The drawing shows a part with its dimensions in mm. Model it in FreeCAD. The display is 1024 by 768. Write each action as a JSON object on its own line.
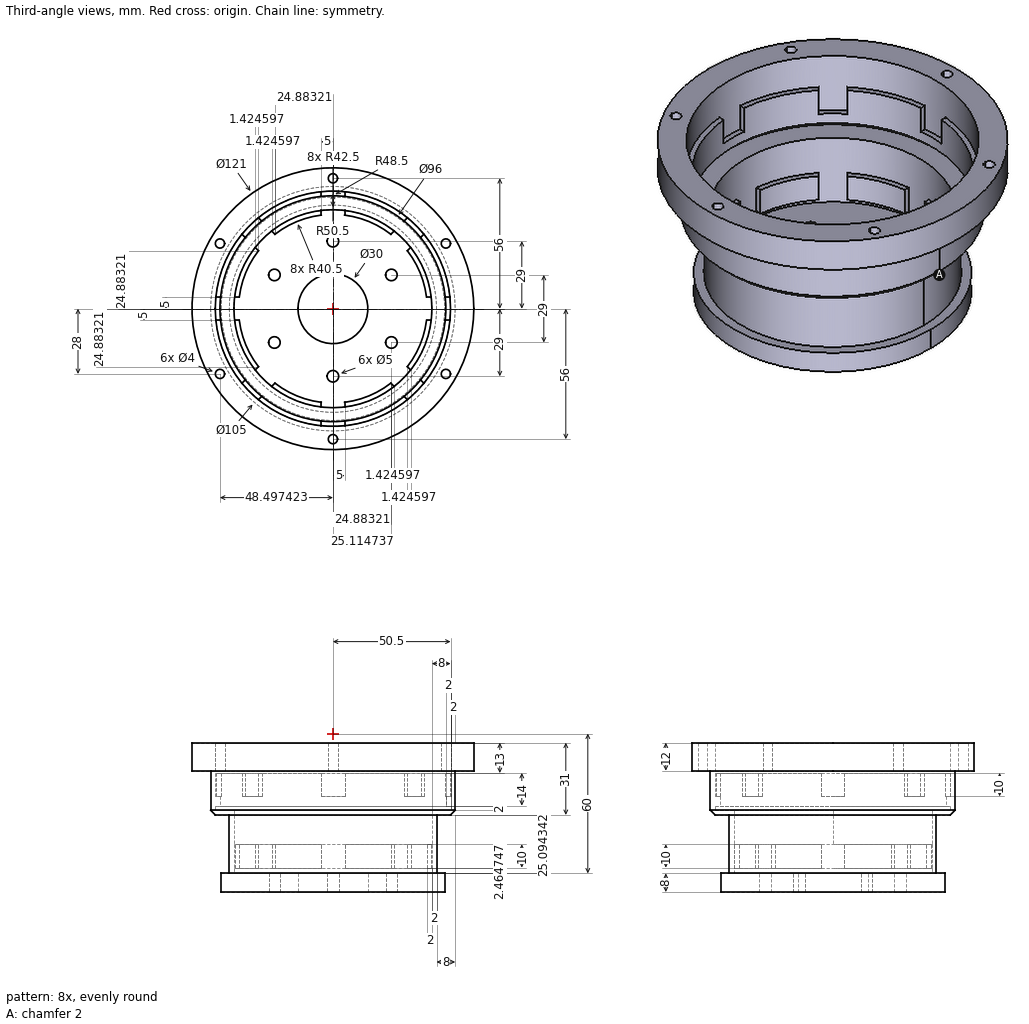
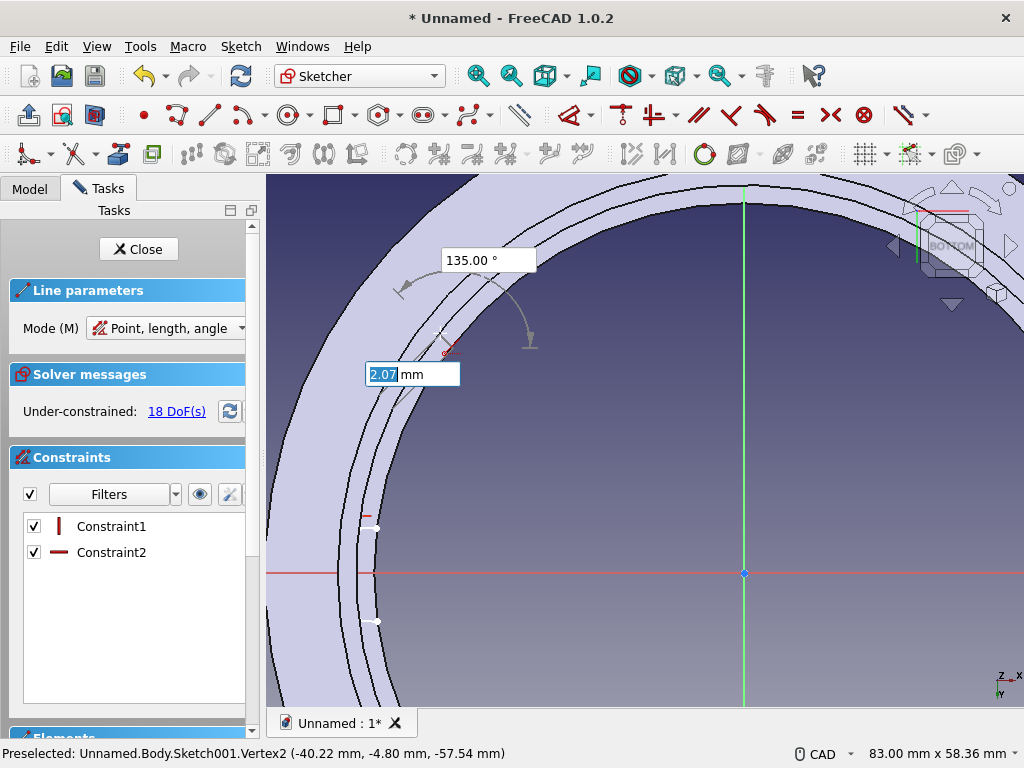
{"action": "left_click", "coordinate": [439, 333]}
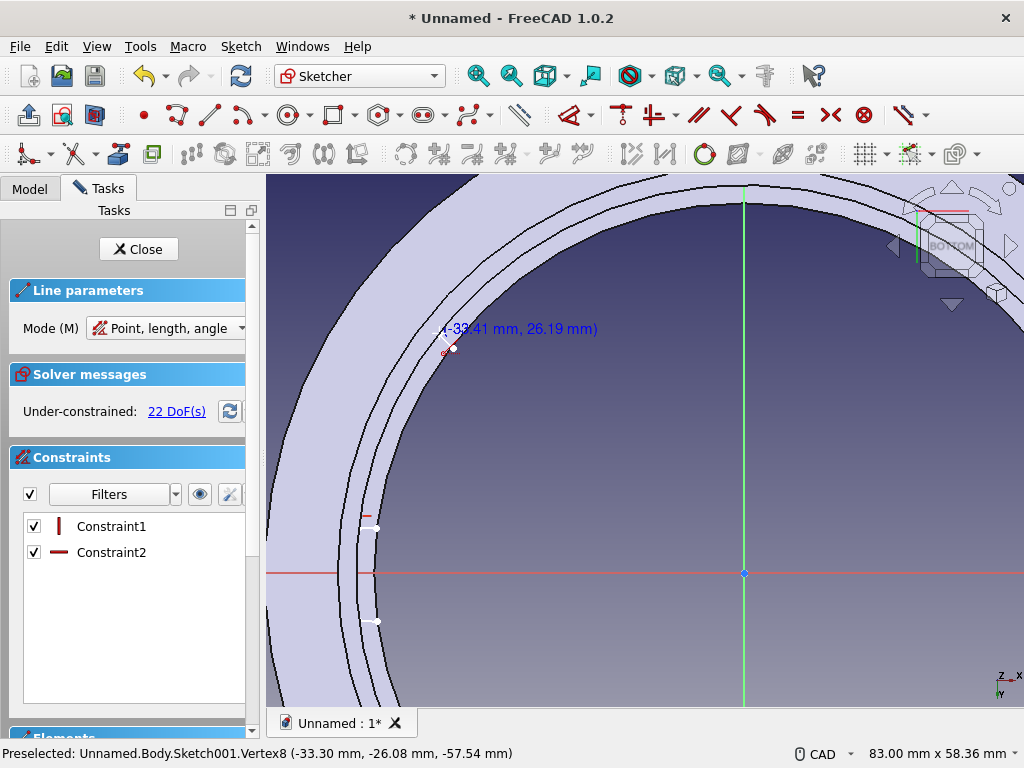
{"action": "left_click", "coordinate": [504, 268]}
{"action": "left_click", "coordinate": [517, 281]}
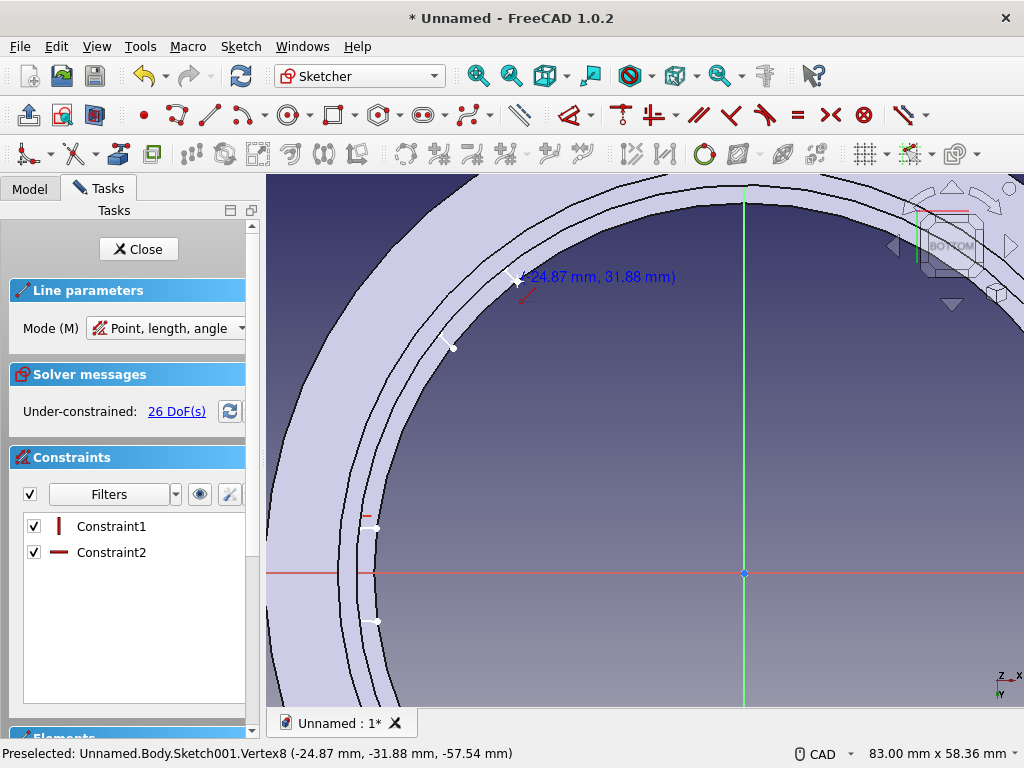
{"action": "left_click", "coordinate": [698, 206]}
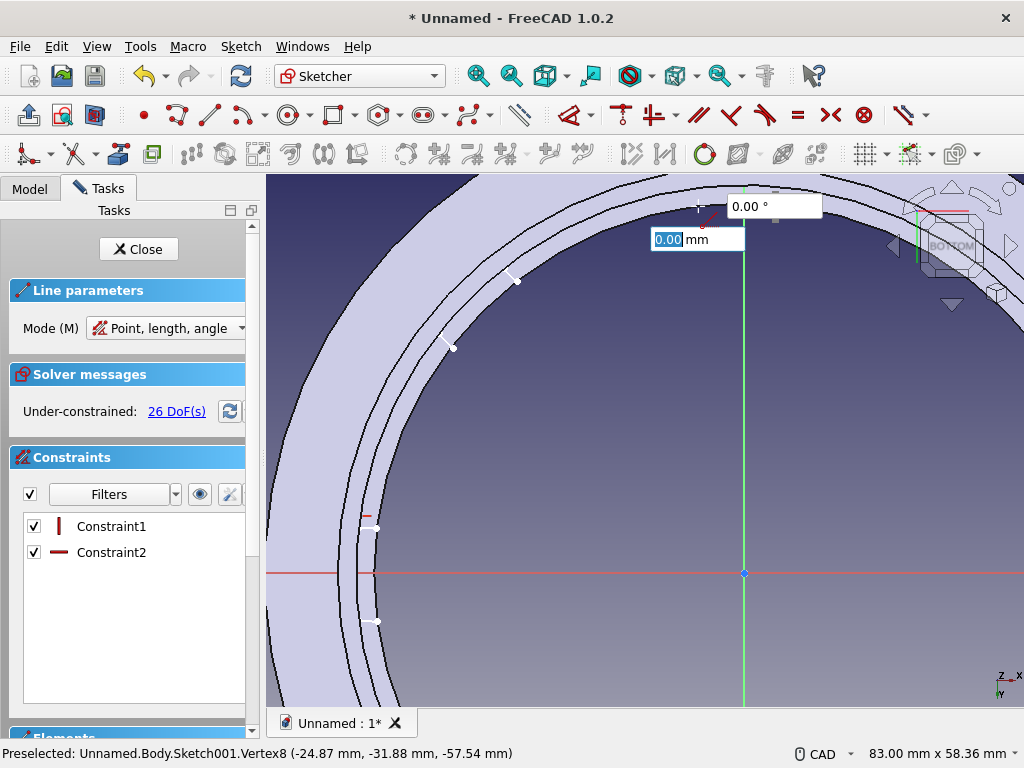
{"action": "scroll", "coordinate": [440, 332], "scroll_direction": "down", "scroll_amount": 4}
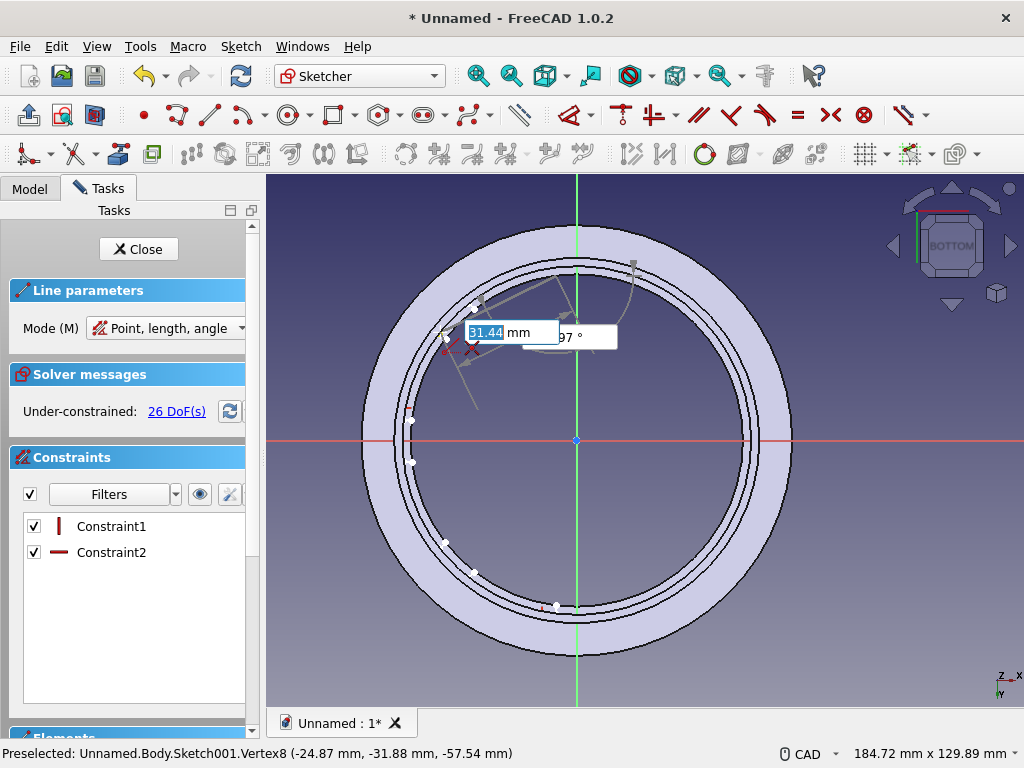
{"action": "scroll", "coordinate": [556, 267], "scroll_direction": "up", "scroll_amount": 4}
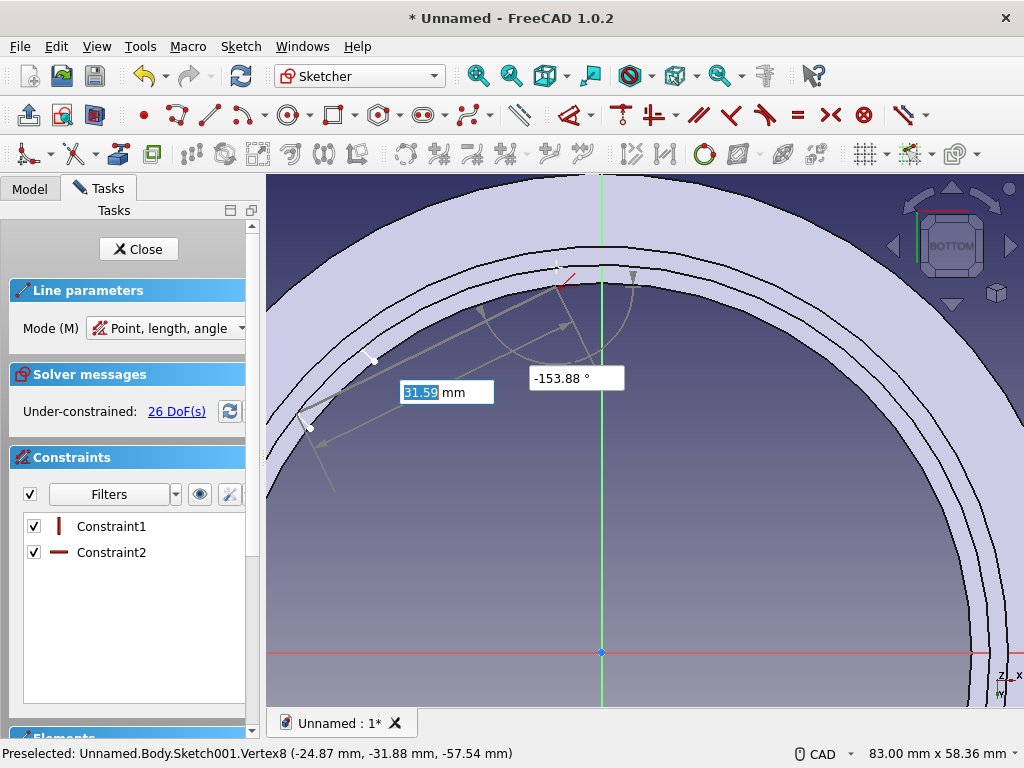
{"action": "left_click", "coordinate": [556, 268]}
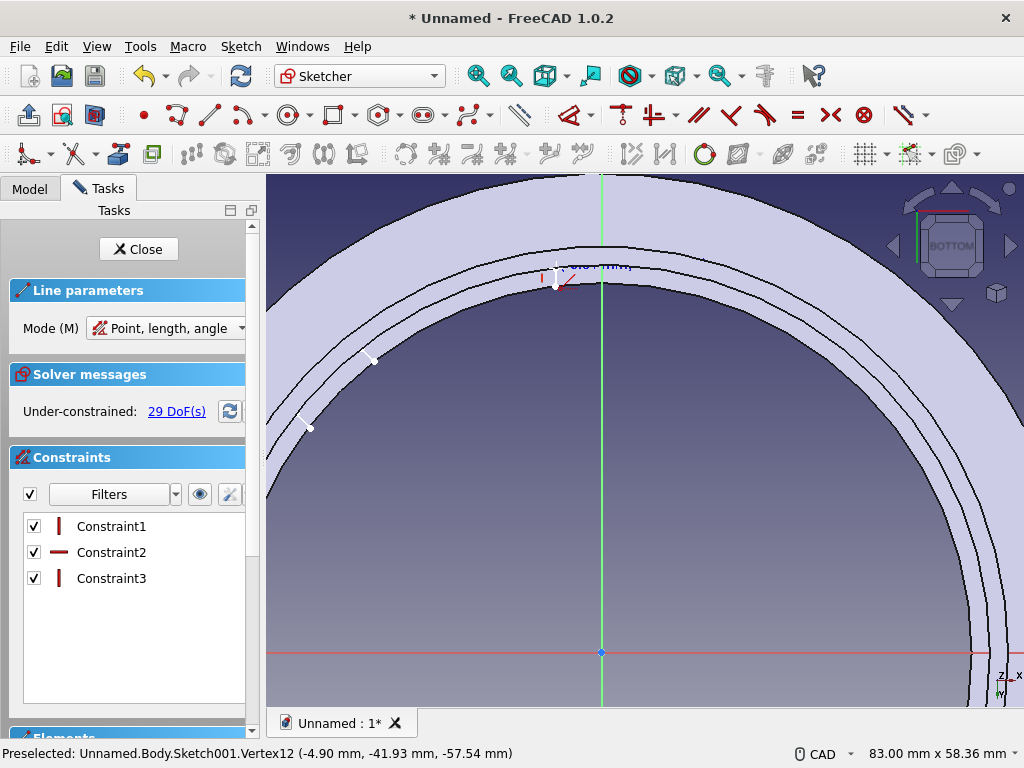
{"action": "left_click", "coordinate": [647, 268]}
{"action": "left_click", "coordinate": [647, 286]}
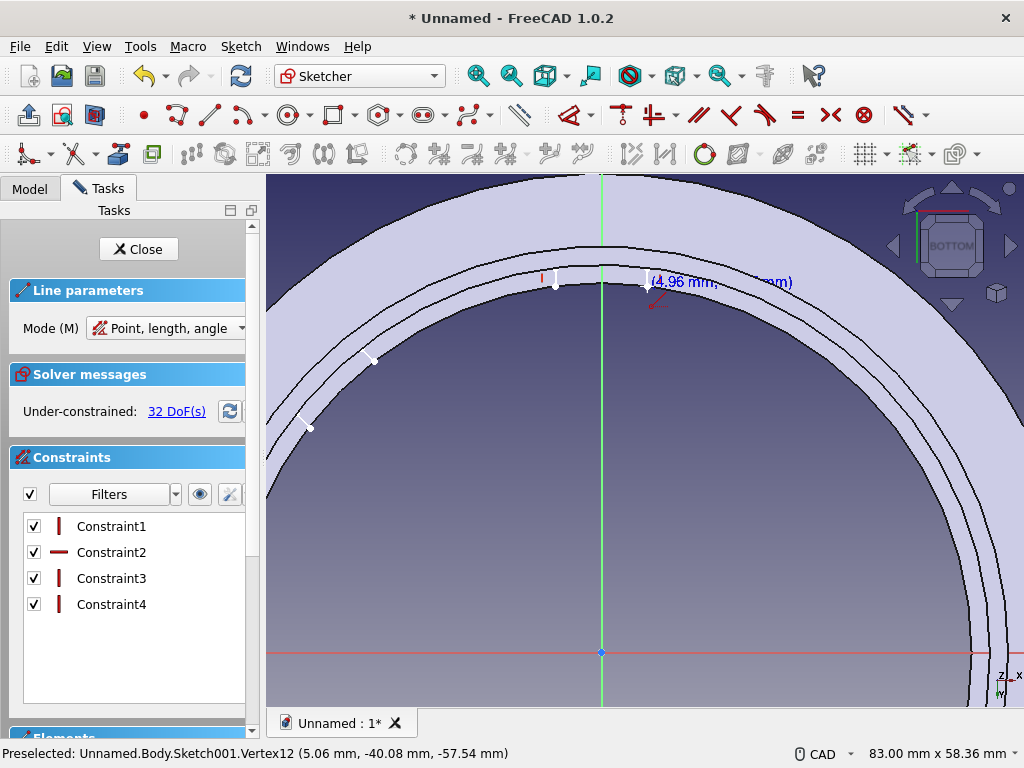
{"action": "left_click", "coordinate": [829, 361]}
{"action": "left_click", "coordinate": [842, 348]}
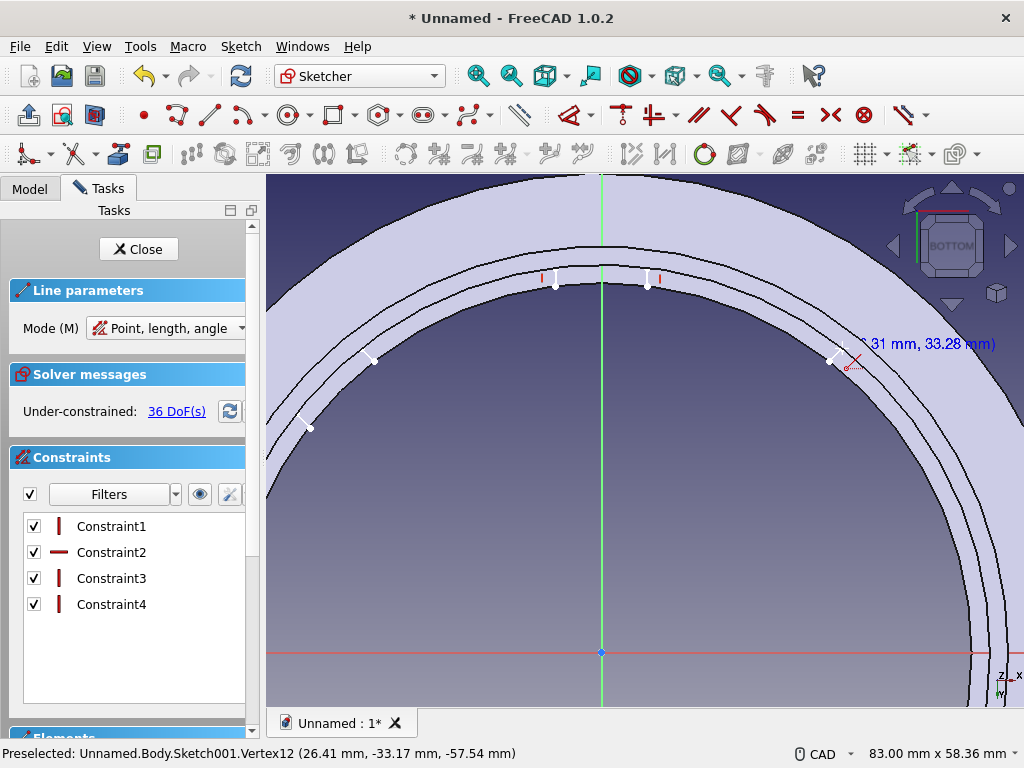
{"action": "scroll", "coordinate": [556, 267], "scroll_direction": "down", "scroll_amount": 4}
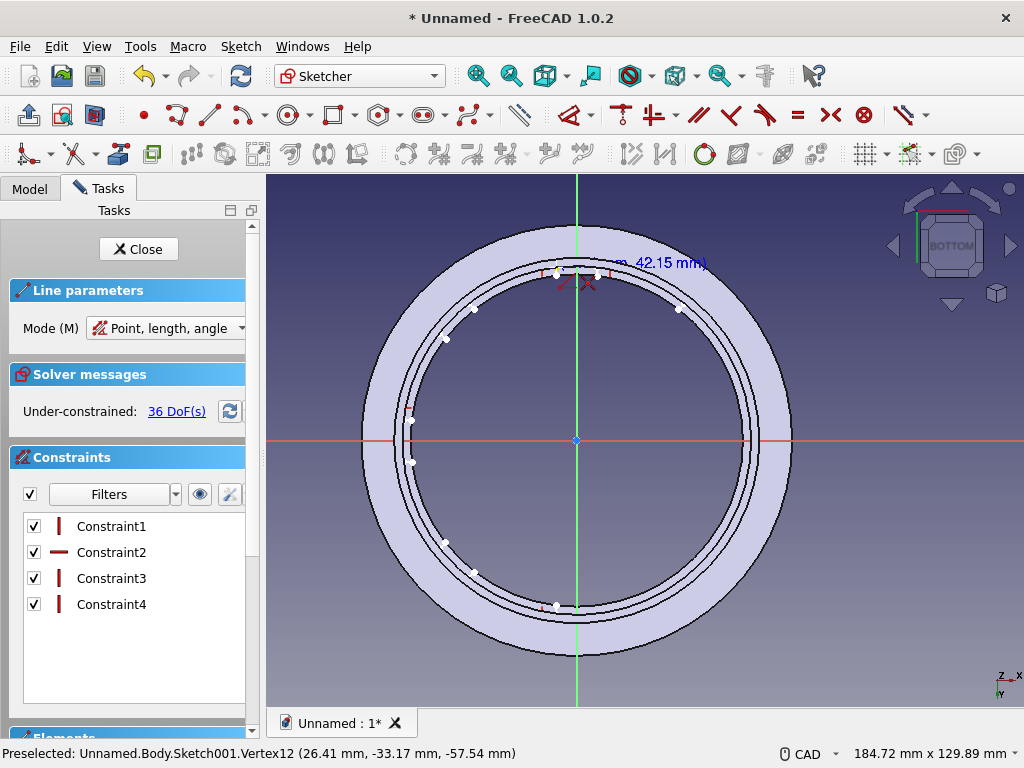
{"action": "left_click", "coordinate": [714, 333]}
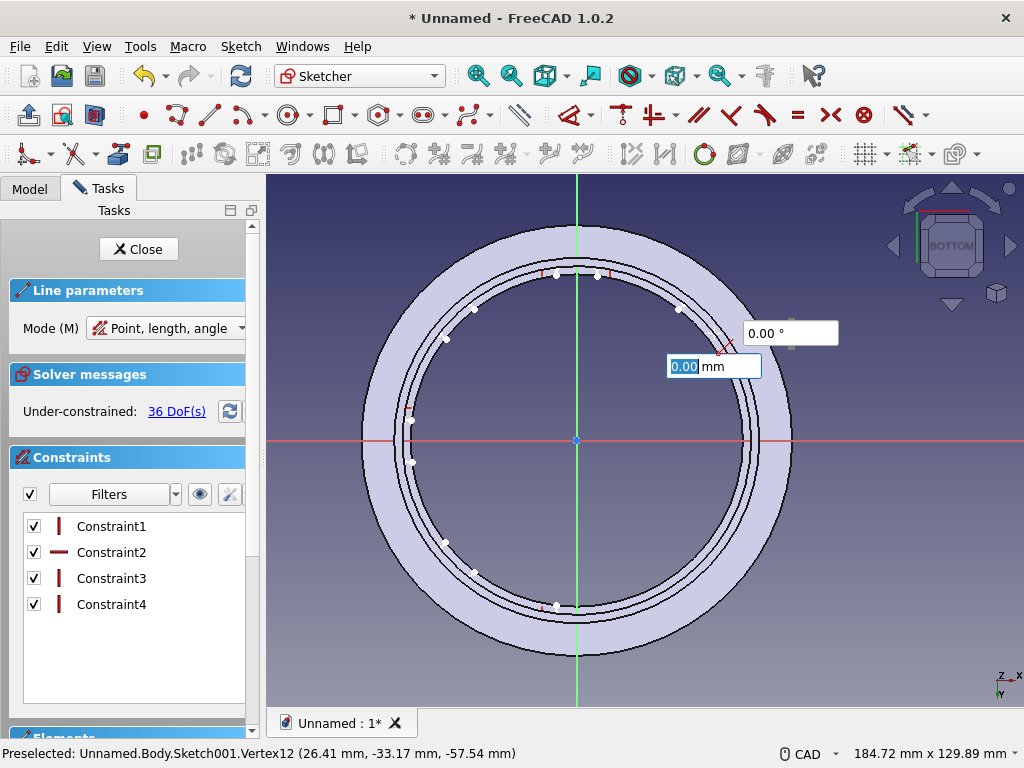
{"action": "scroll", "coordinate": [708, 338], "scroll_direction": "up", "scroll_amount": 4}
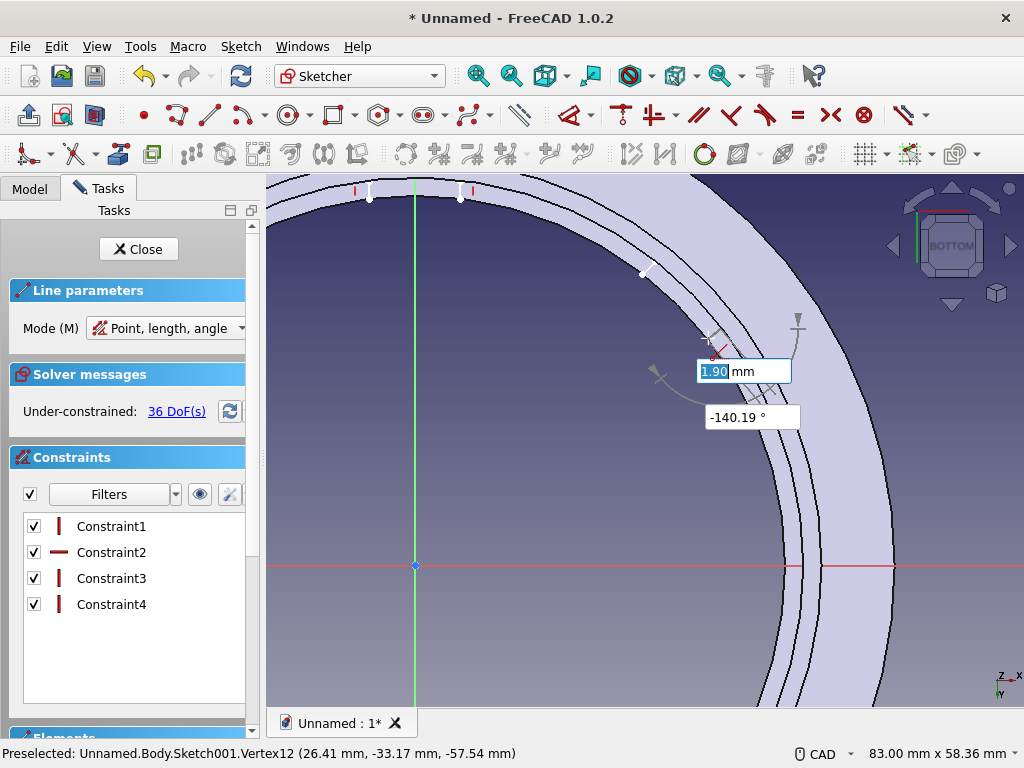
{"action": "left_click", "coordinate": [707, 339]}